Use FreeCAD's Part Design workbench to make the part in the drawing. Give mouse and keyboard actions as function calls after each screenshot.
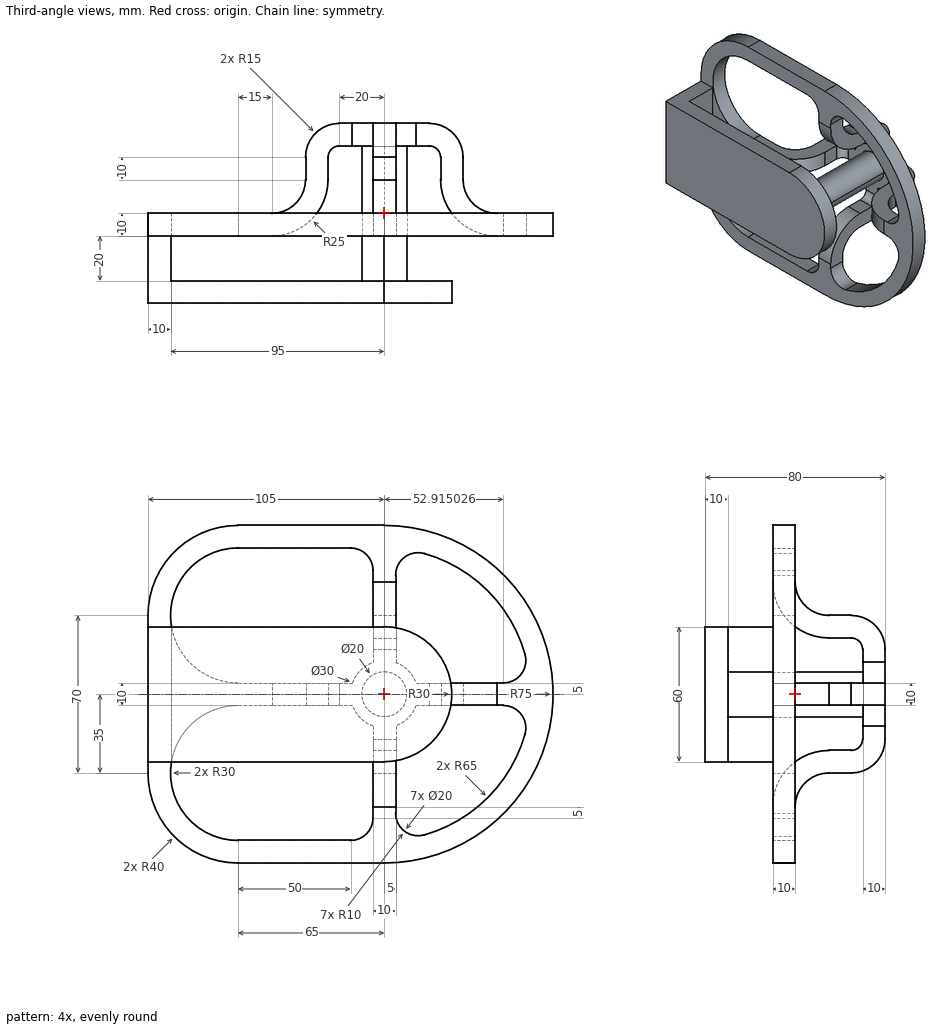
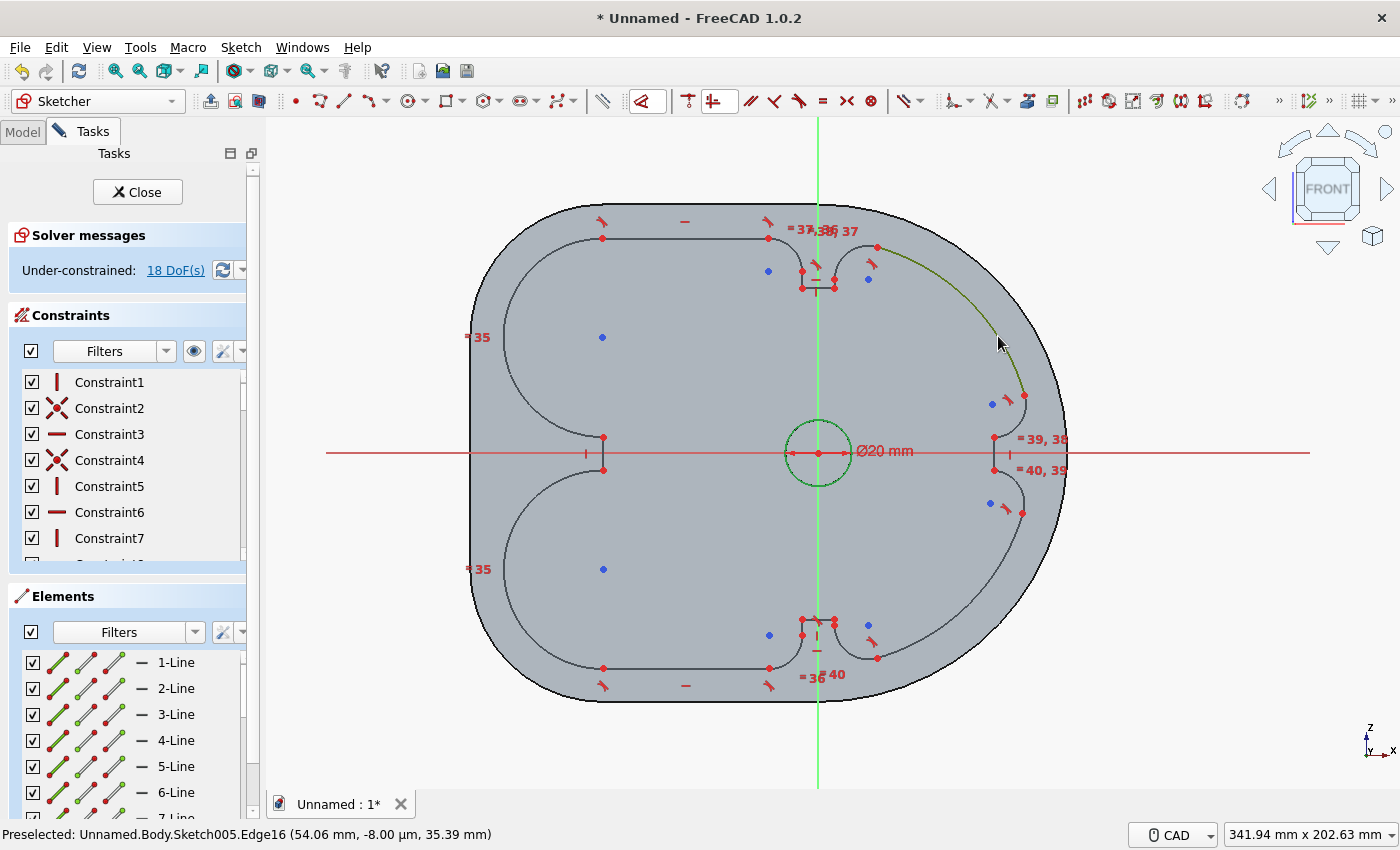
click(936, 631)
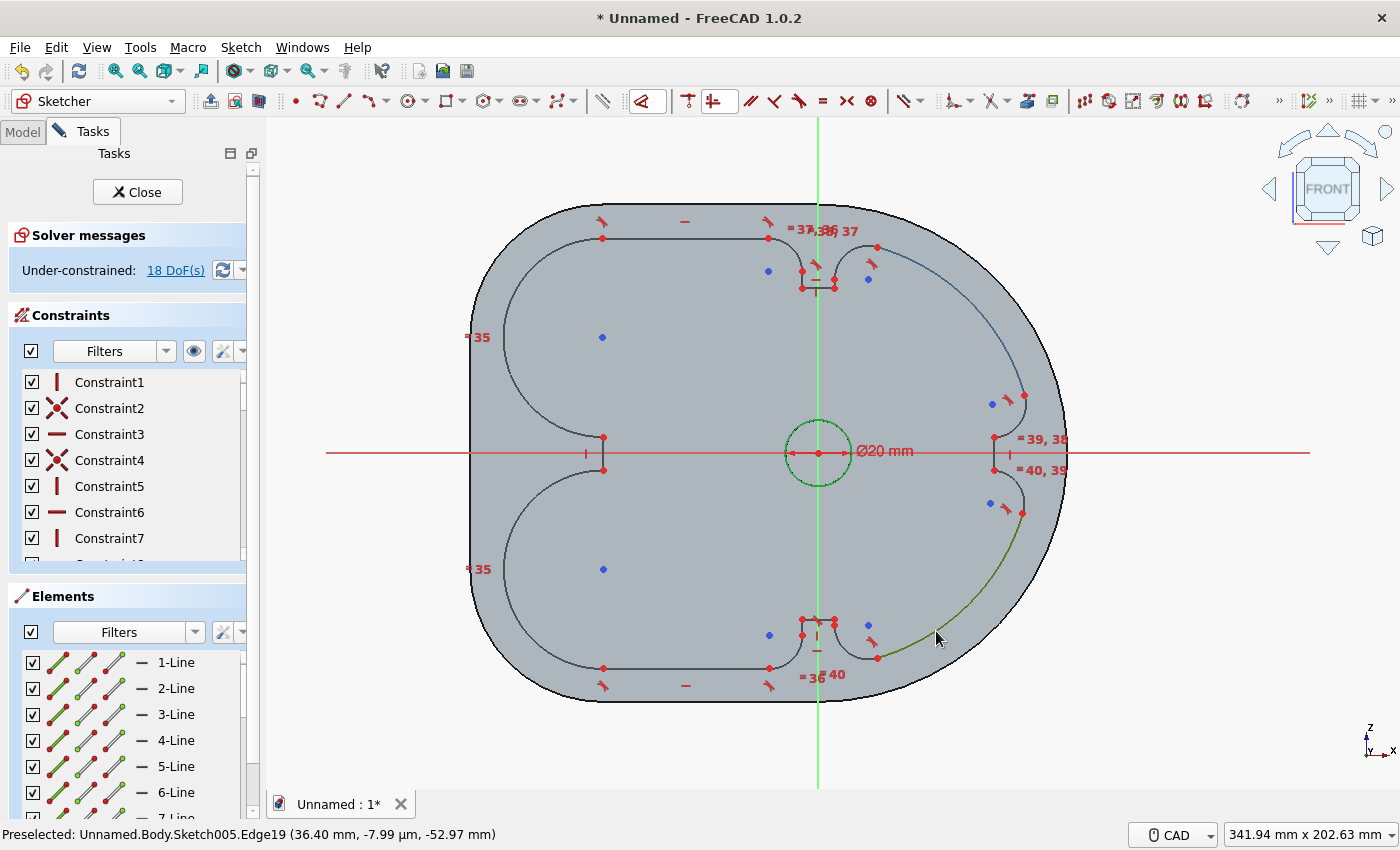
click(824, 102)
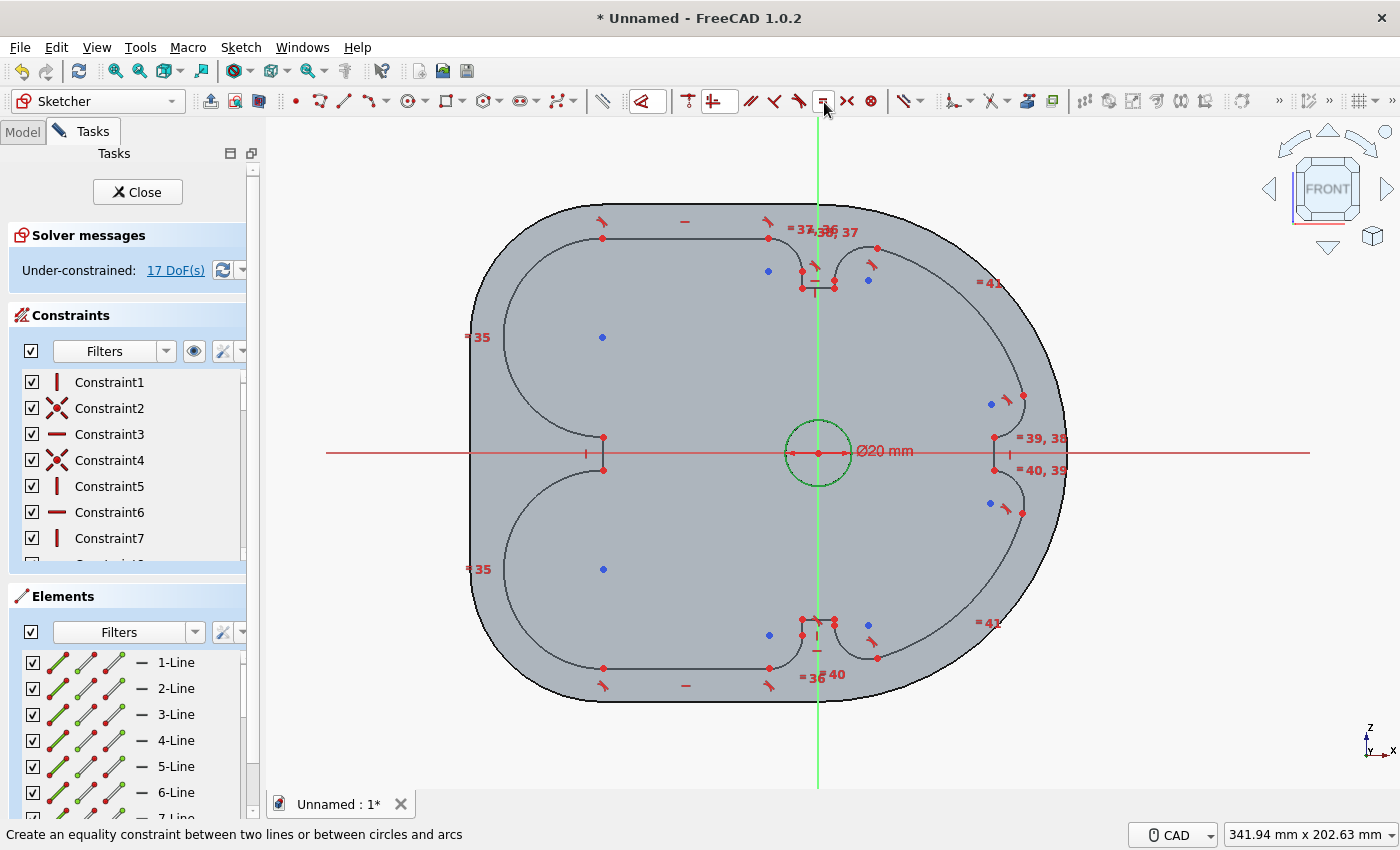
click(603, 570)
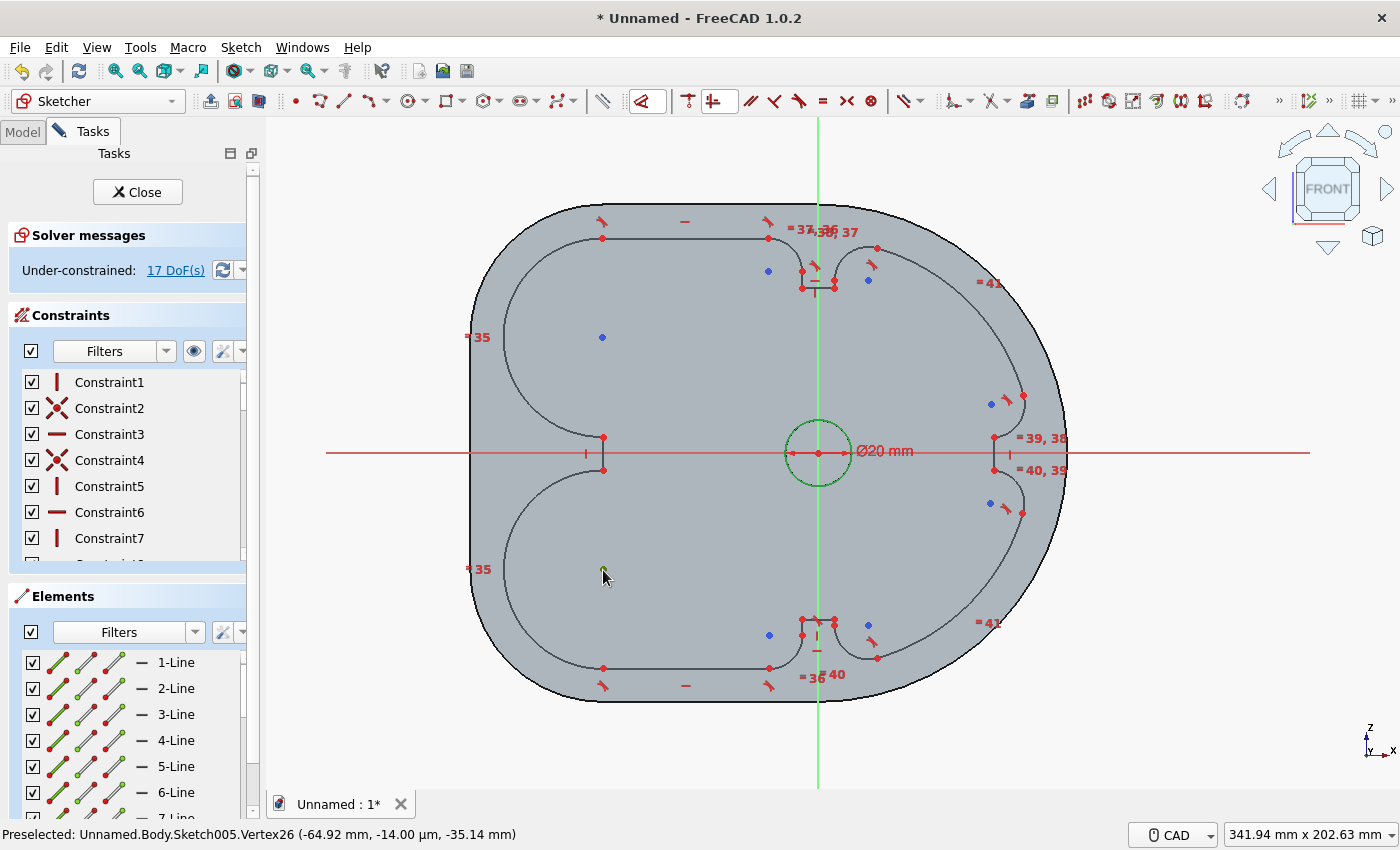
click(603, 338)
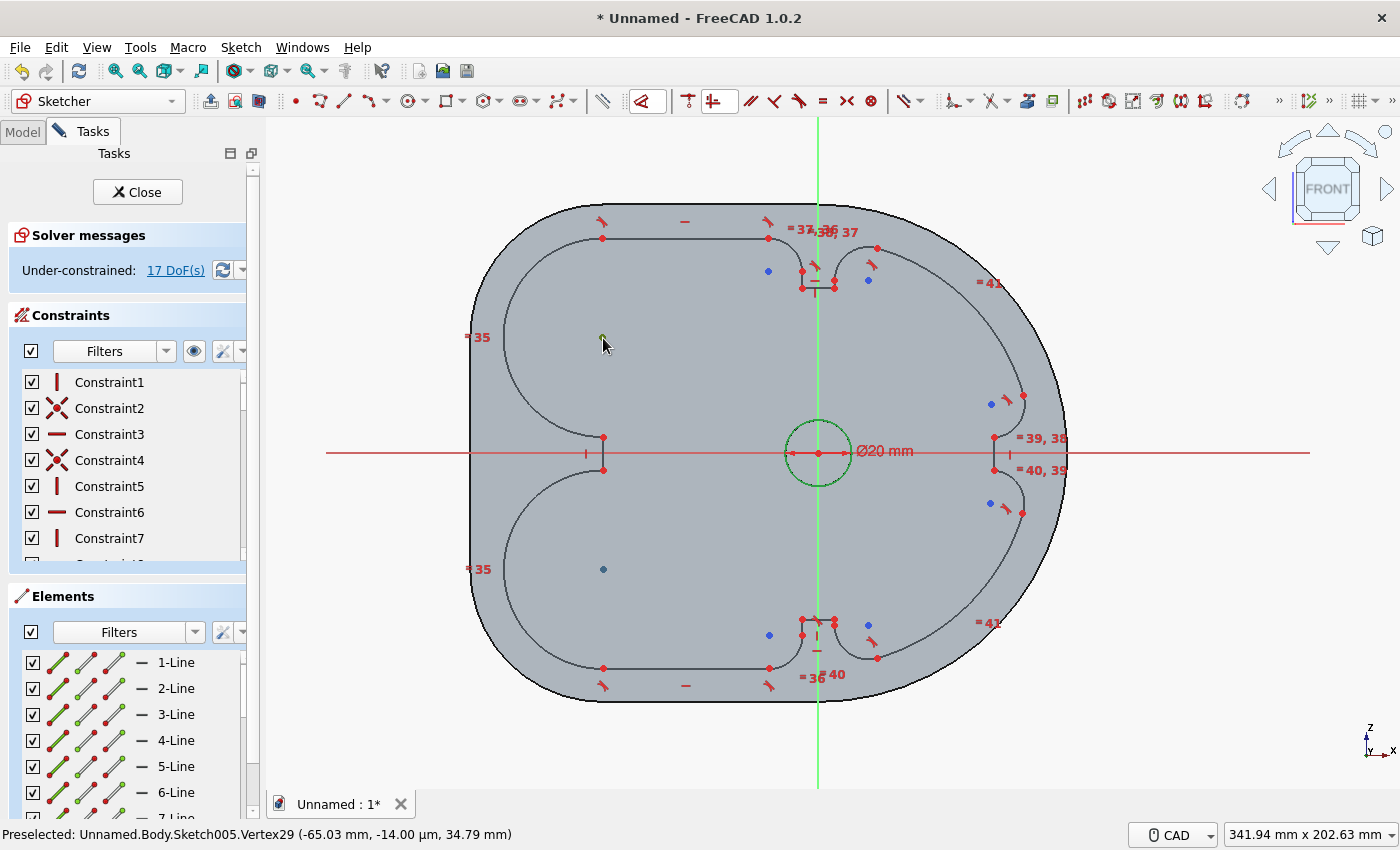
click(361, 453)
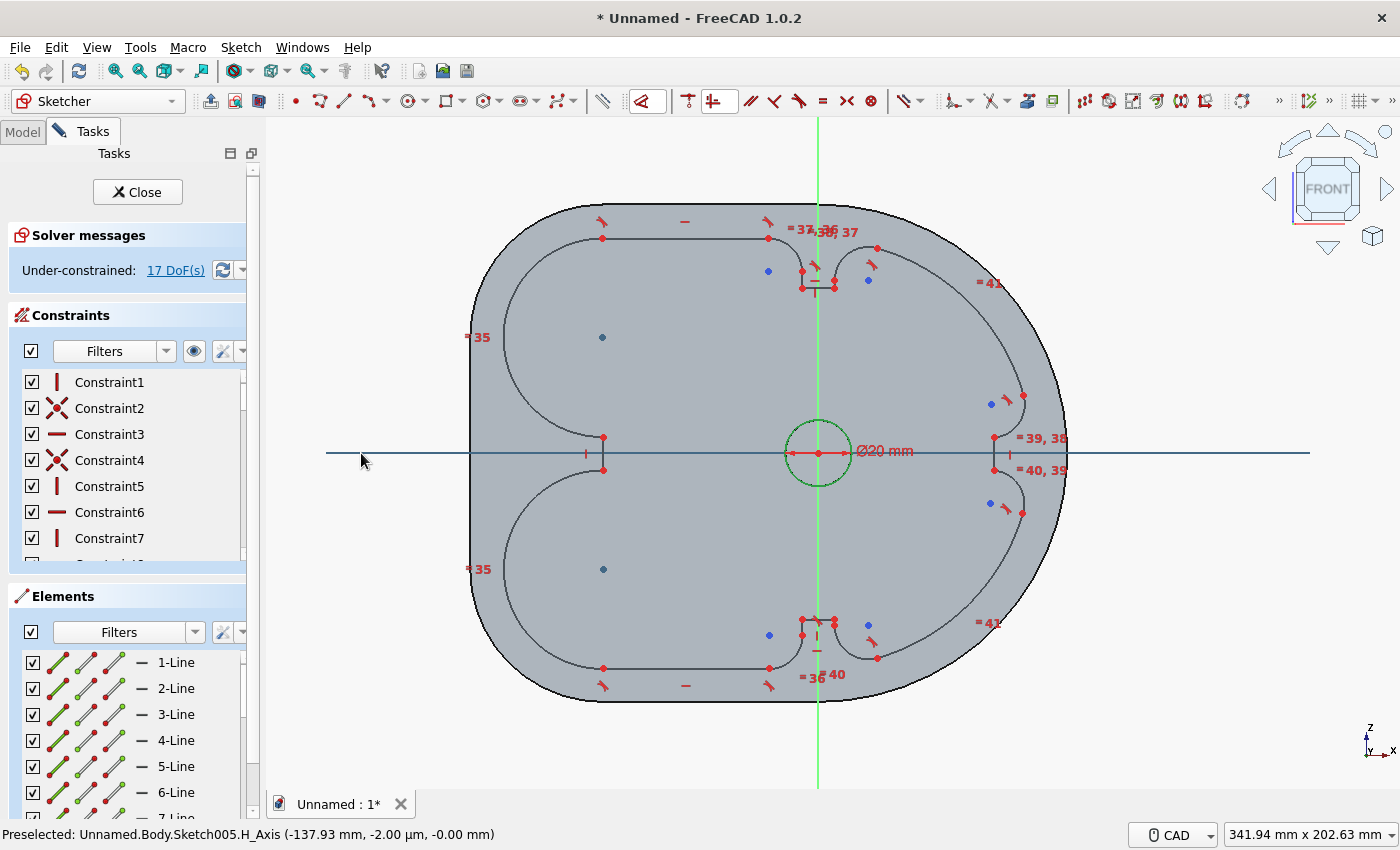
click(848, 102)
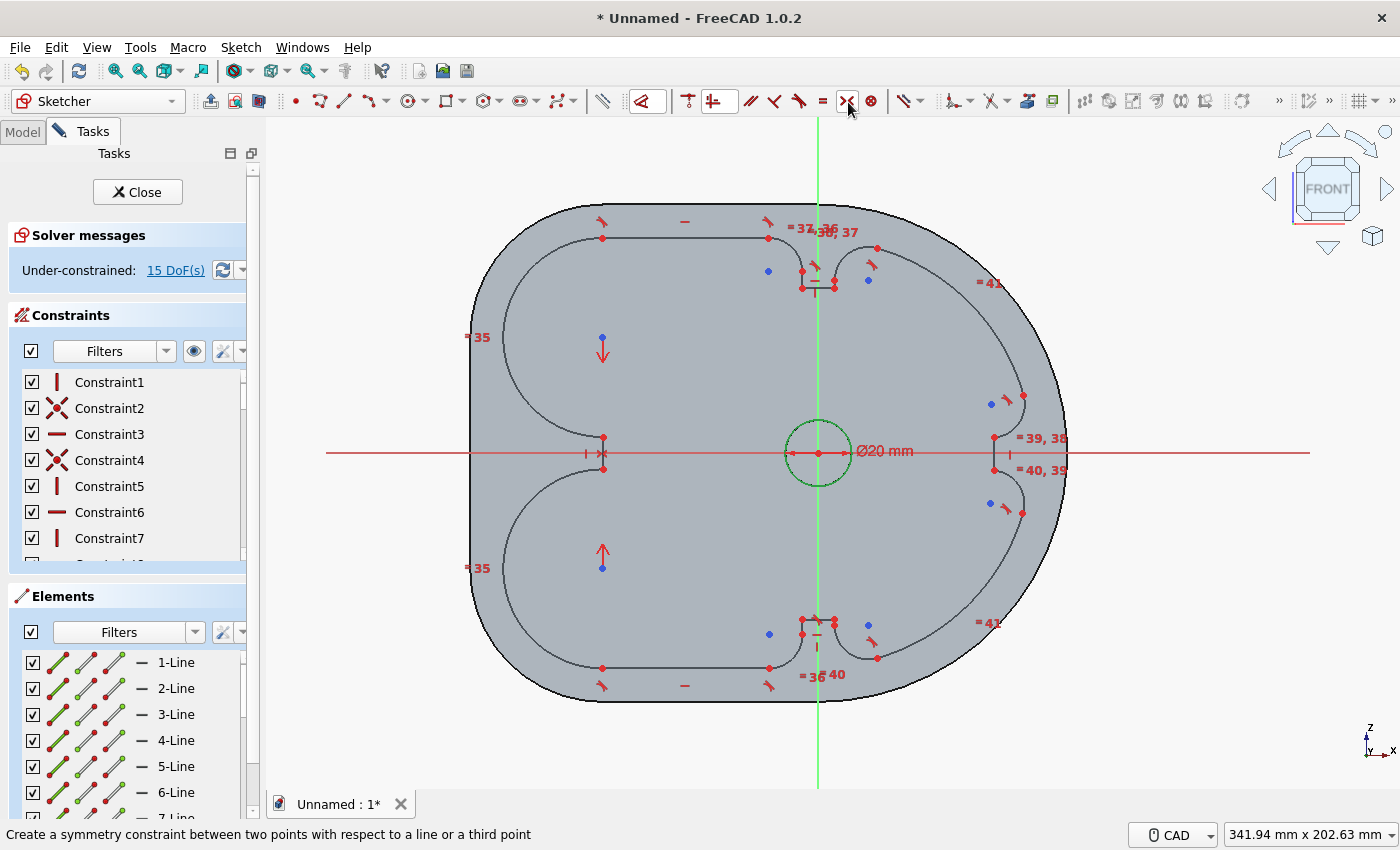
click(802, 620)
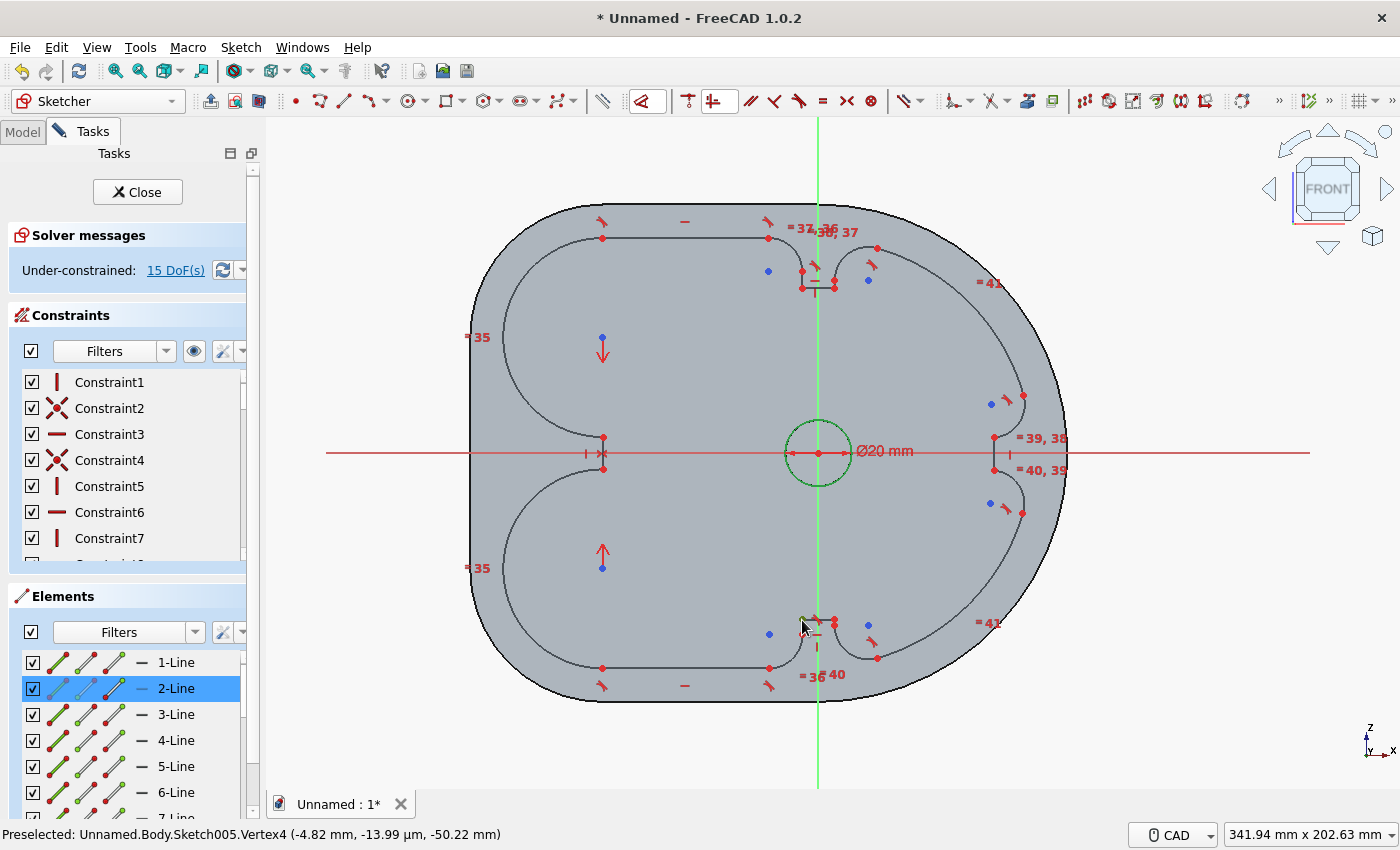
click(802, 288)